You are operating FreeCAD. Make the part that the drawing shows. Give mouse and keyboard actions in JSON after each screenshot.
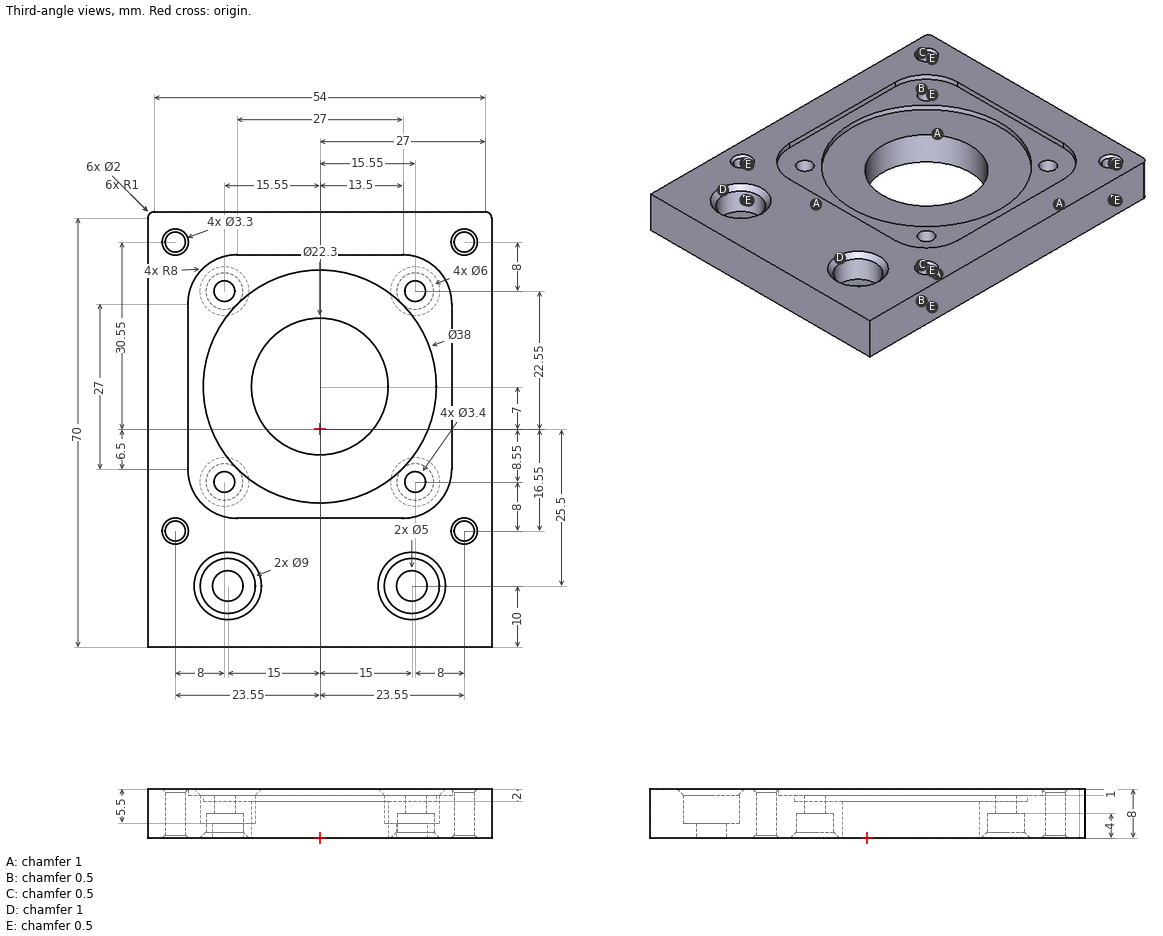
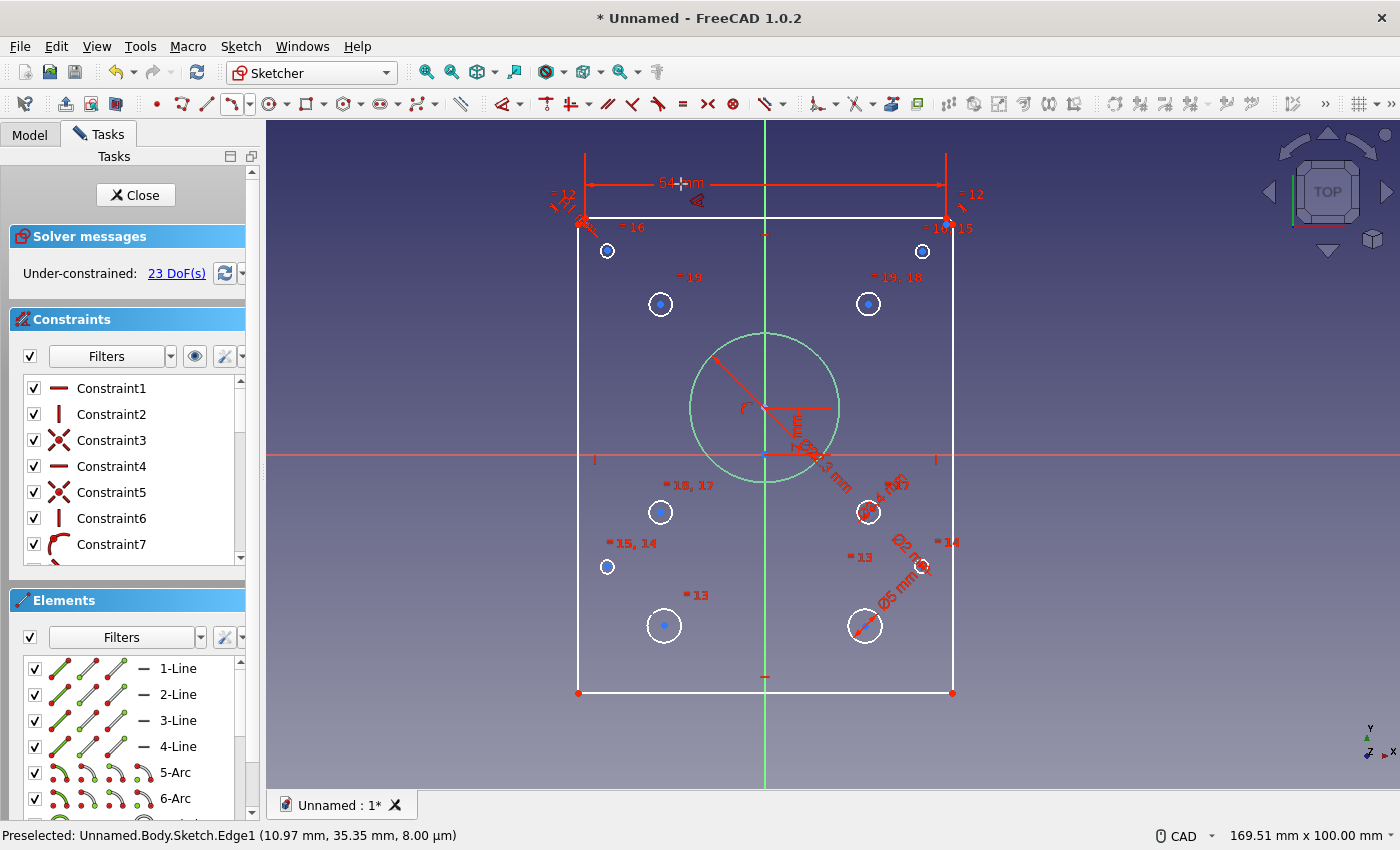
{"action": "left_click", "coordinate": [578, 365]}
{"action": "left_click", "coordinate": [544, 351]}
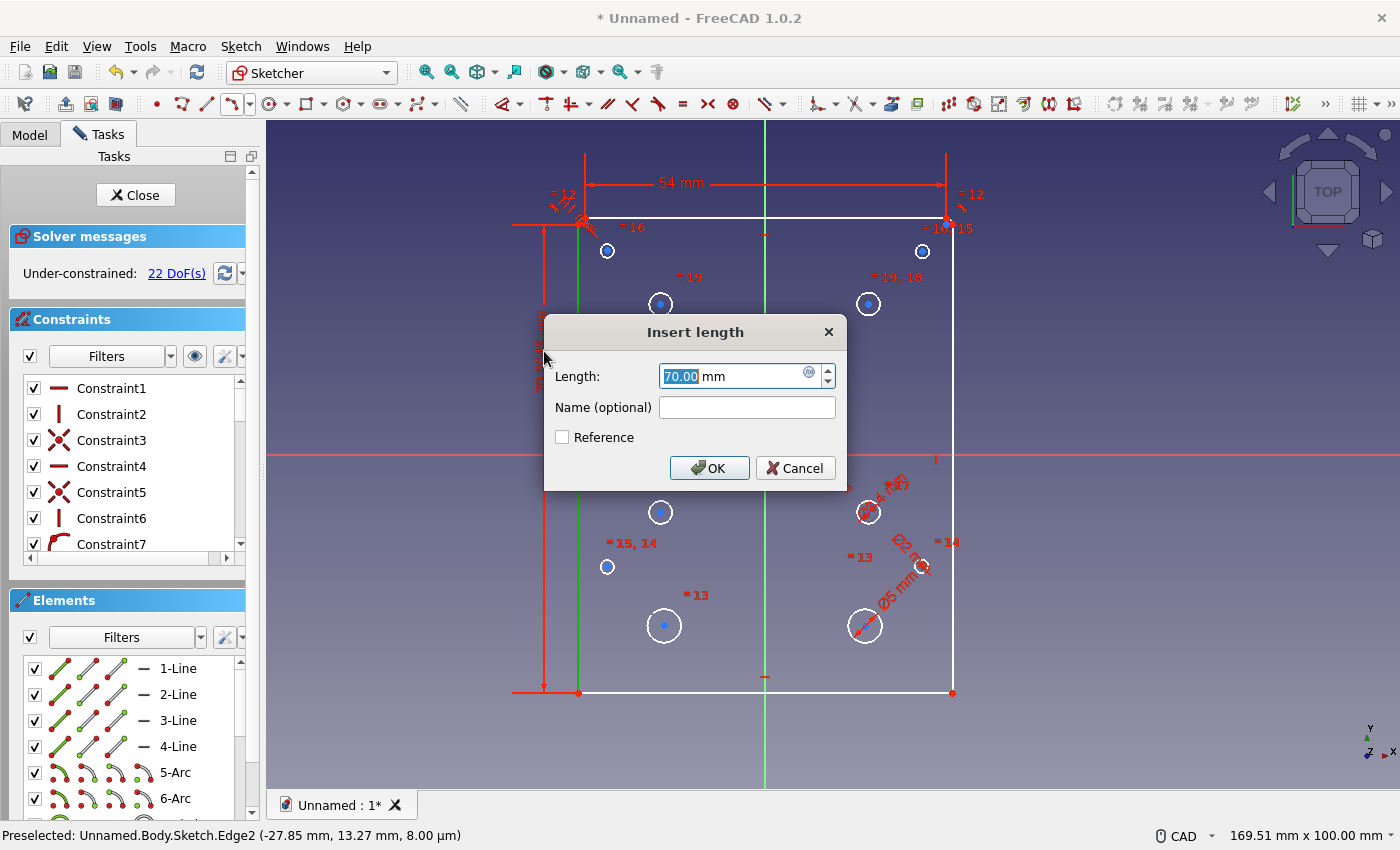
{"action": "type", "text": "70"}
{"action": "key", "text": "Return"}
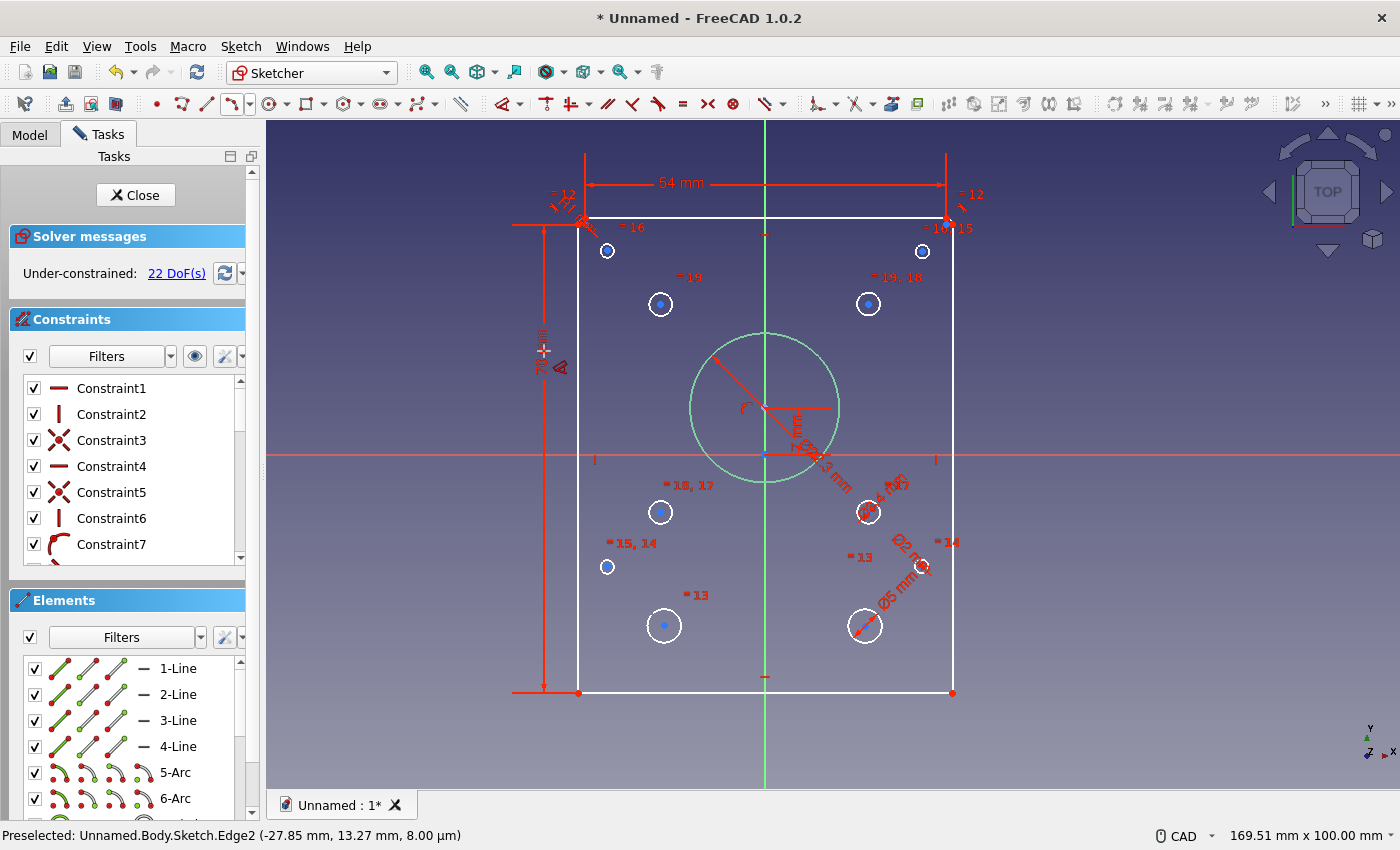
{"action": "left_click", "coordinate": [865, 626]}
{"action": "left_click", "coordinate": [815, 660]}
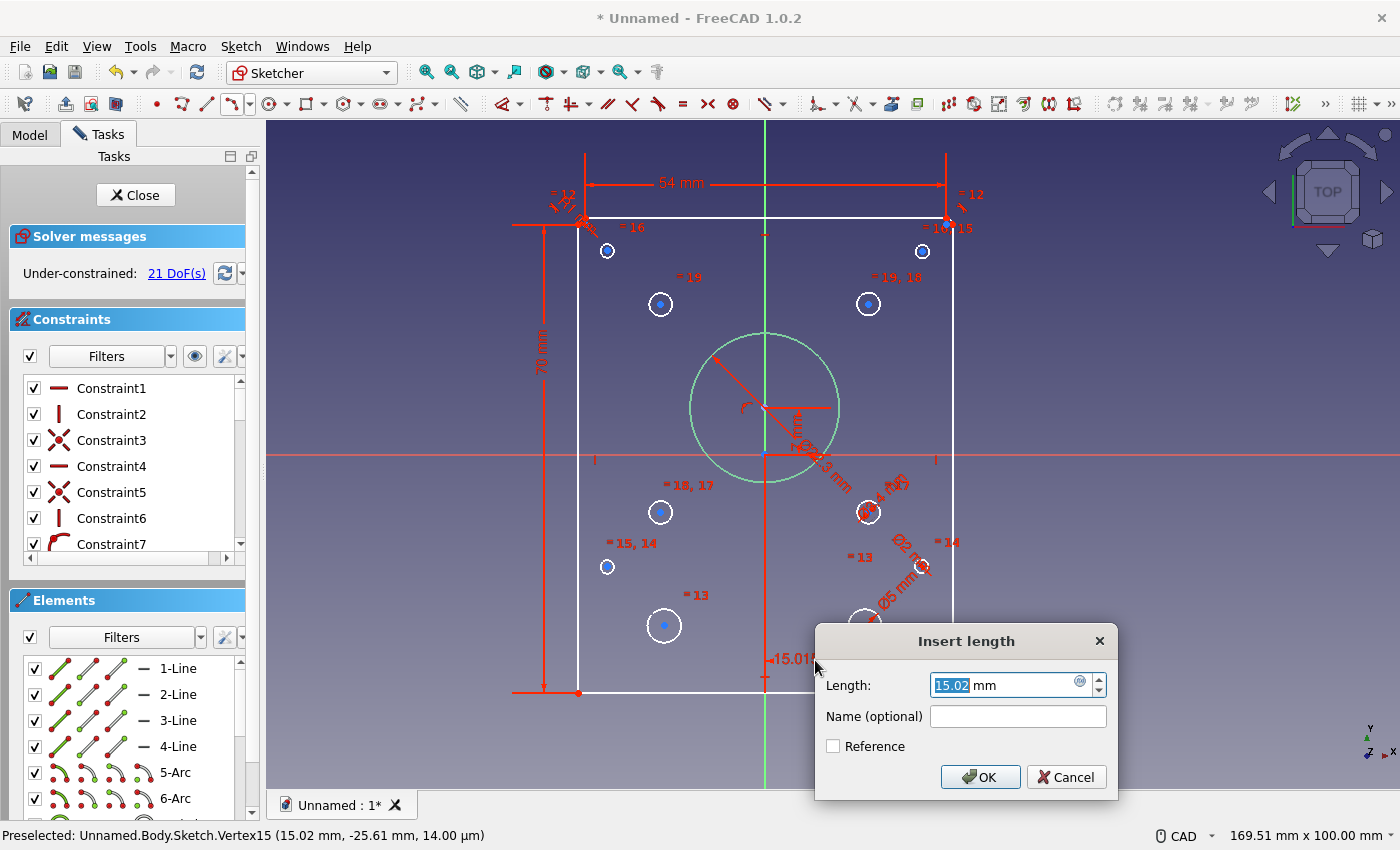
{"action": "type", "text": "15"}
{"action": "key", "text": "Return"}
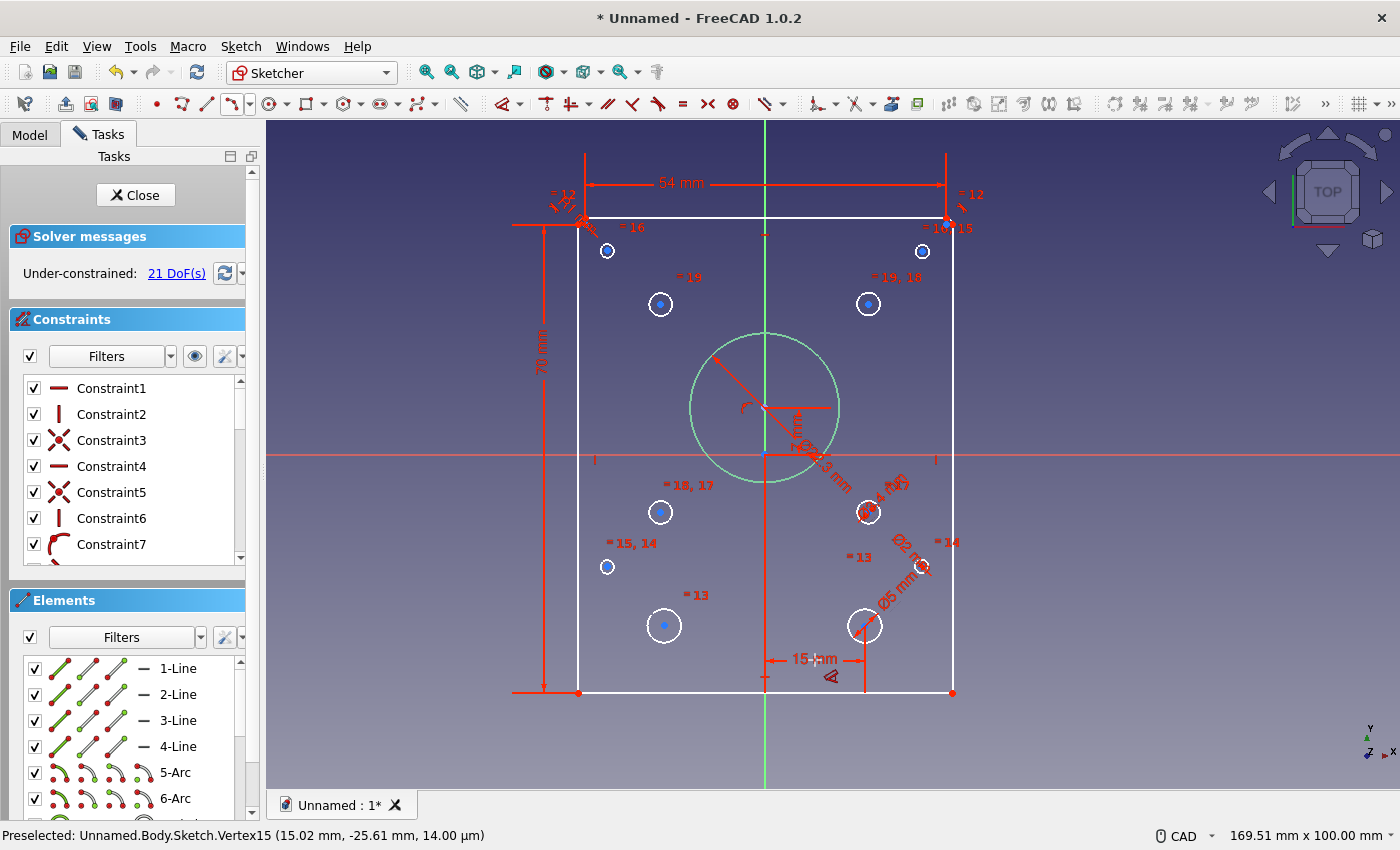
{"action": "left_click", "coordinate": [664, 626]}
{"action": "left_click", "coordinate": [714, 660]}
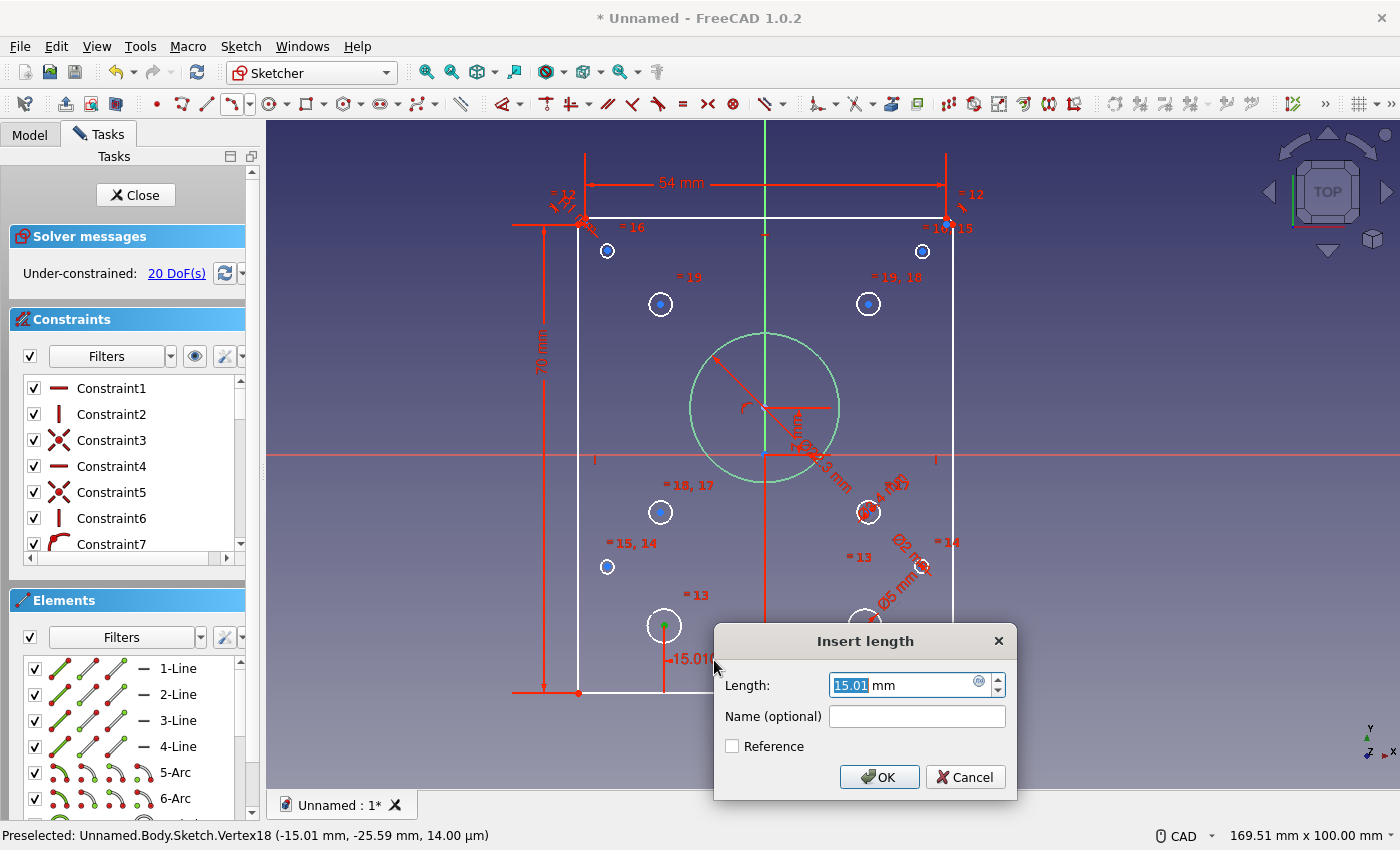
{"action": "type", "text": "15"}
{"action": "key", "text": "Return"}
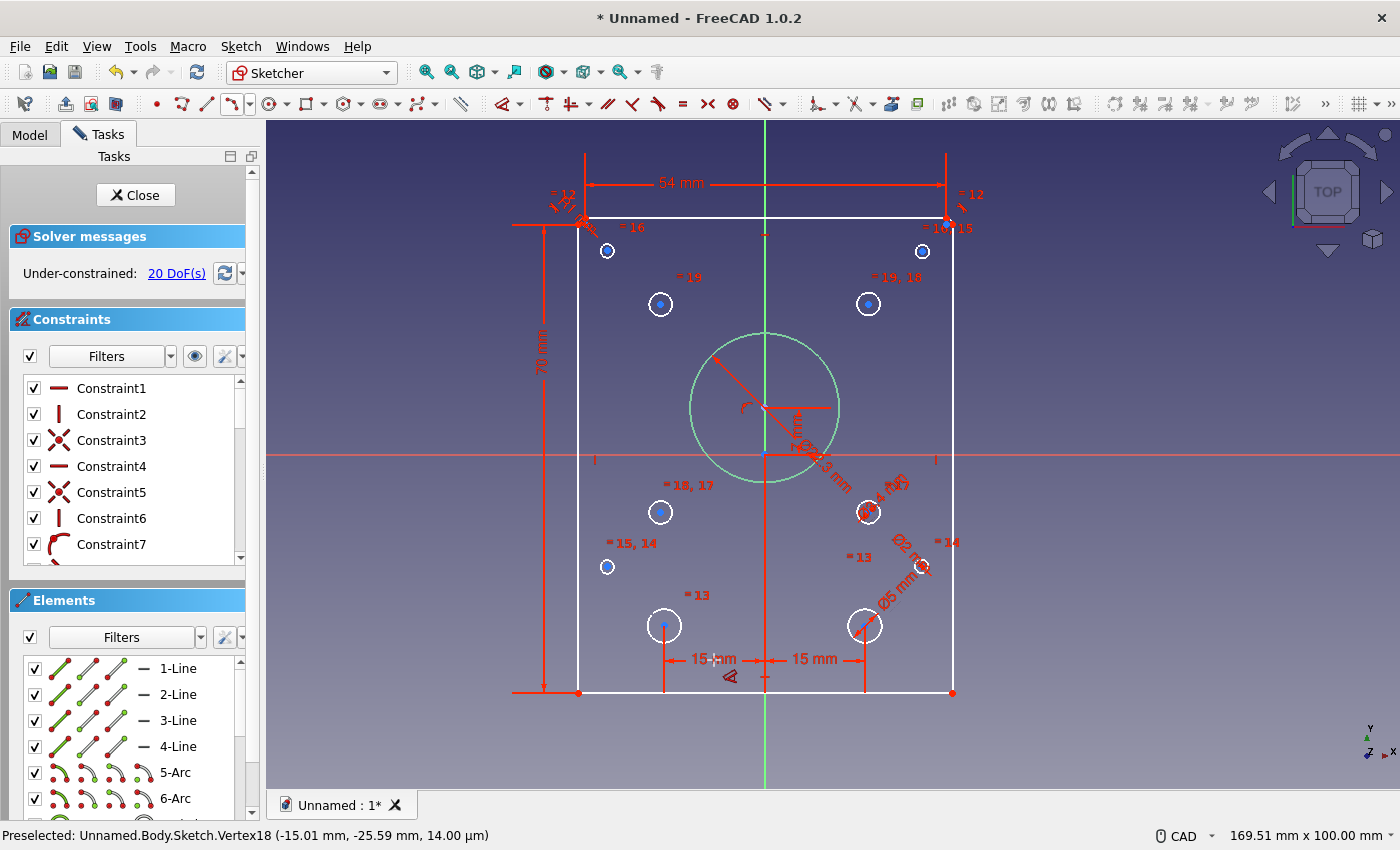
{"action": "left_click", "coordinate": [922, 566]}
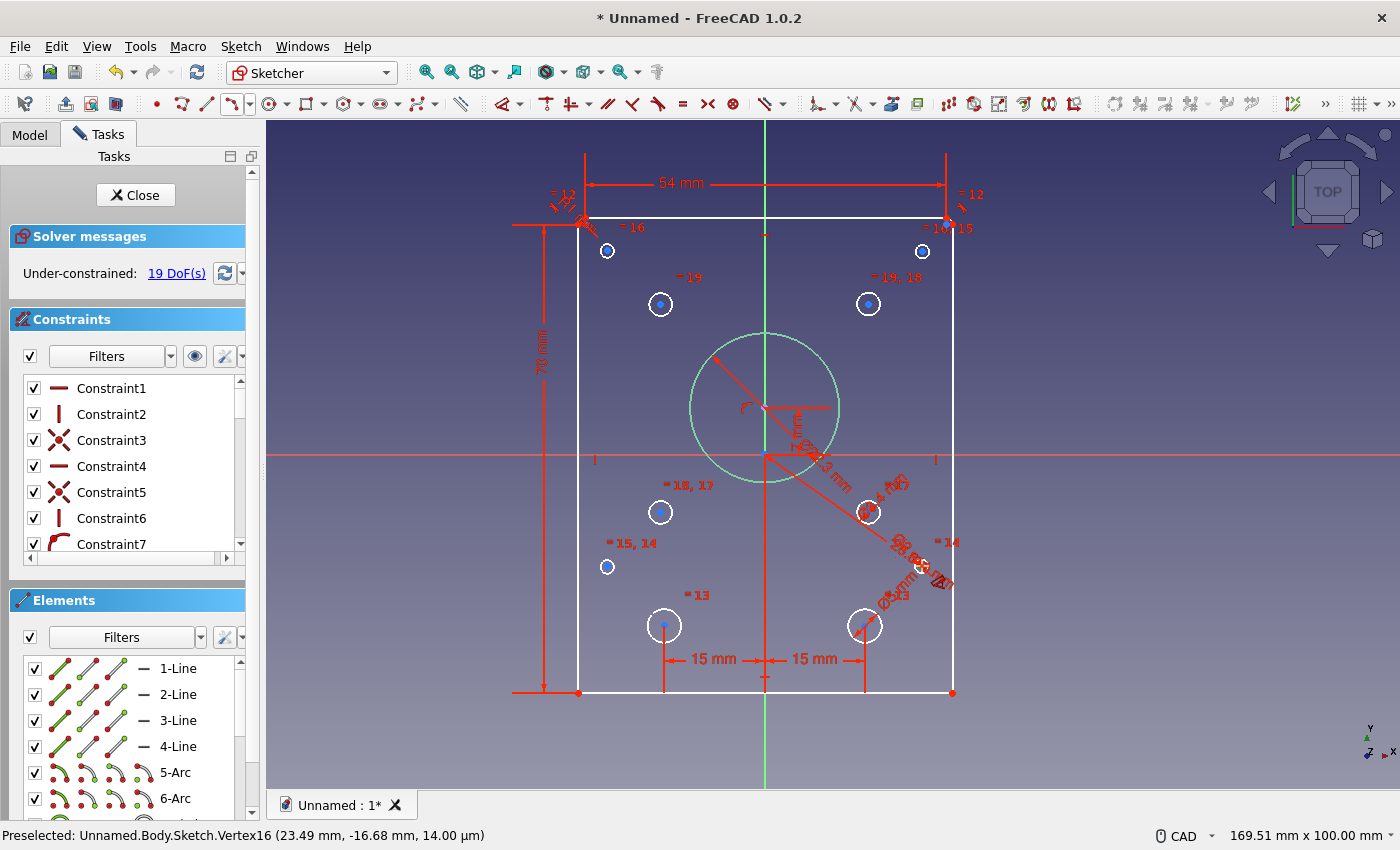
{"action": "left_click", "coordinate": [869, 512]}
{"action": "left_click", "coordinate": [895, 624]}